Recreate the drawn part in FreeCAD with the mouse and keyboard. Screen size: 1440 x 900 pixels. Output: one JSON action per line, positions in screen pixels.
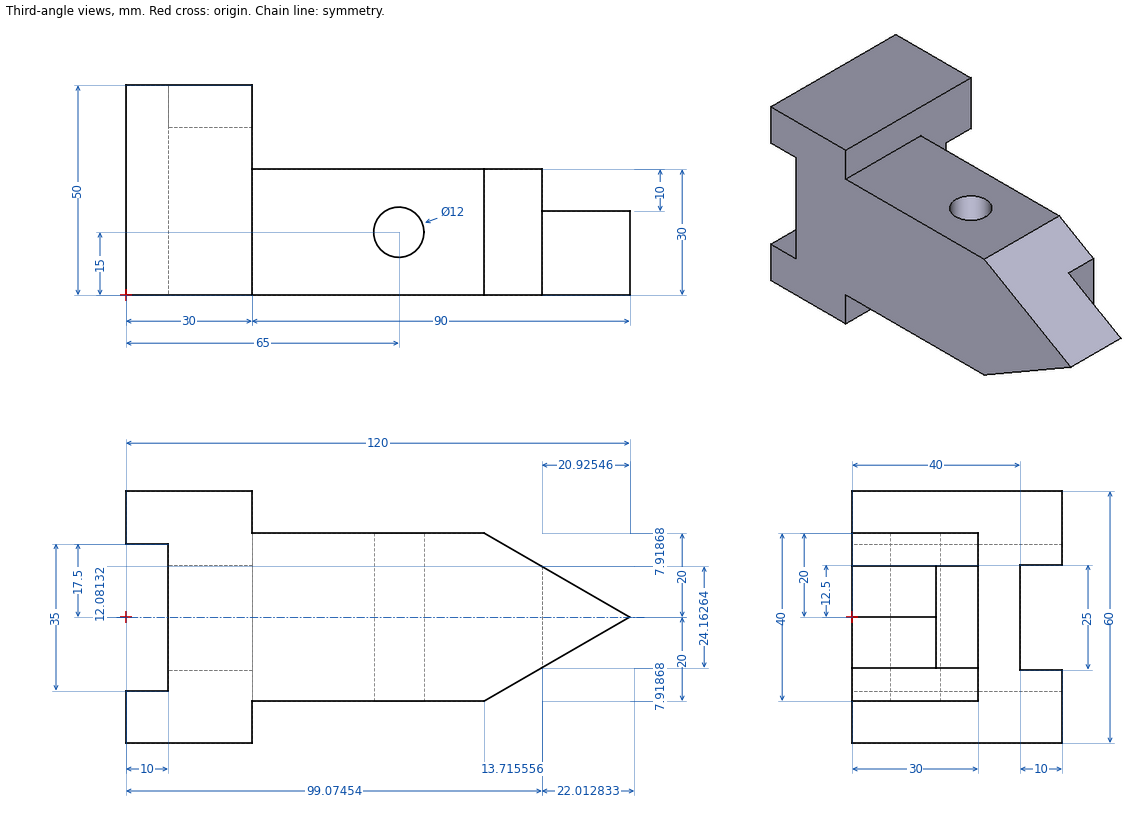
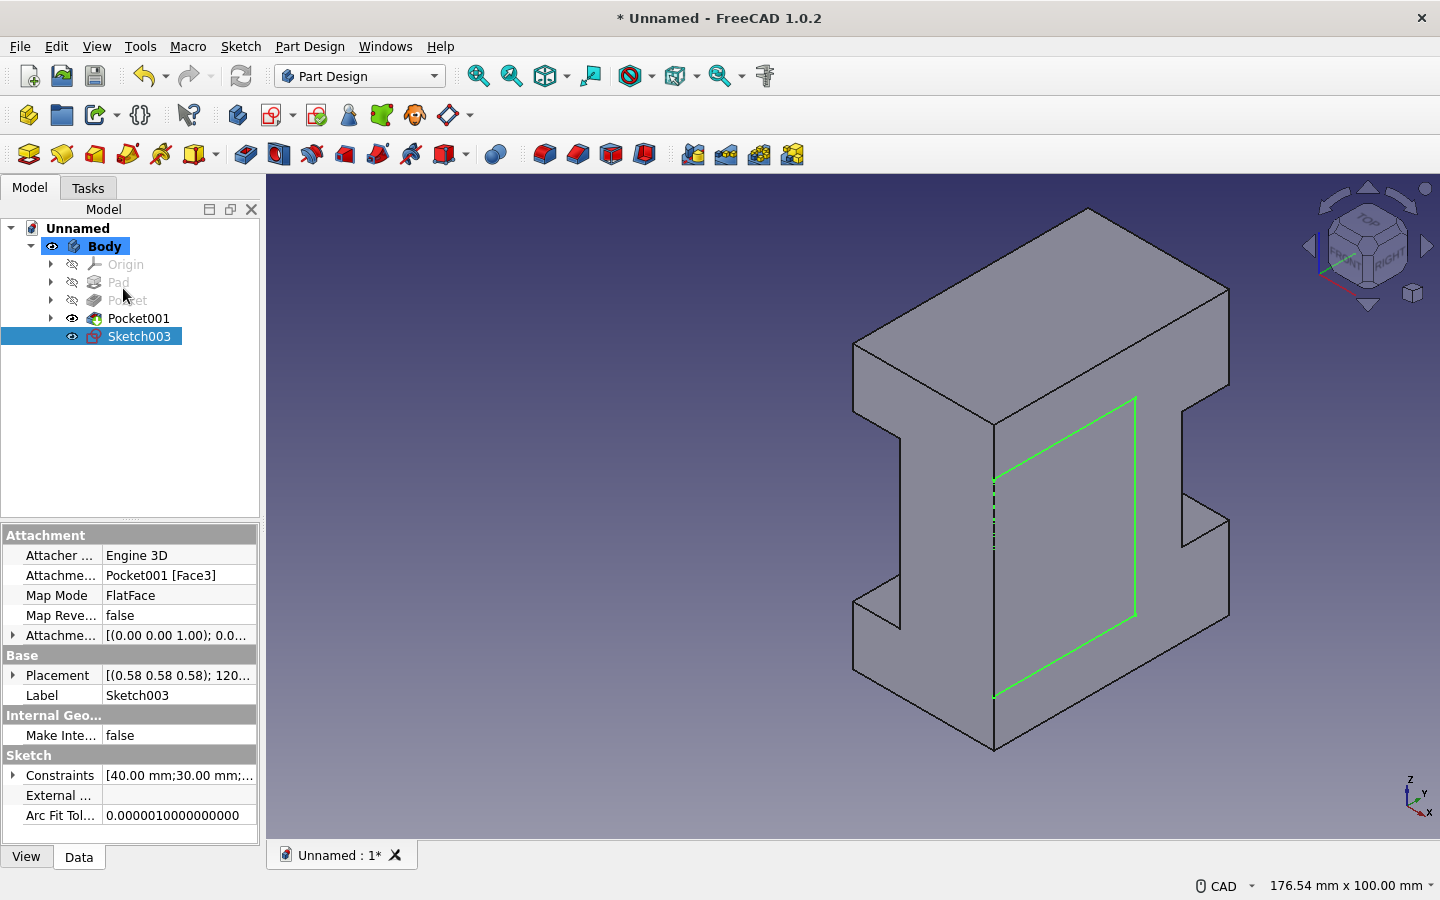
{"action": "left_click", "coordinate": [29, 154]}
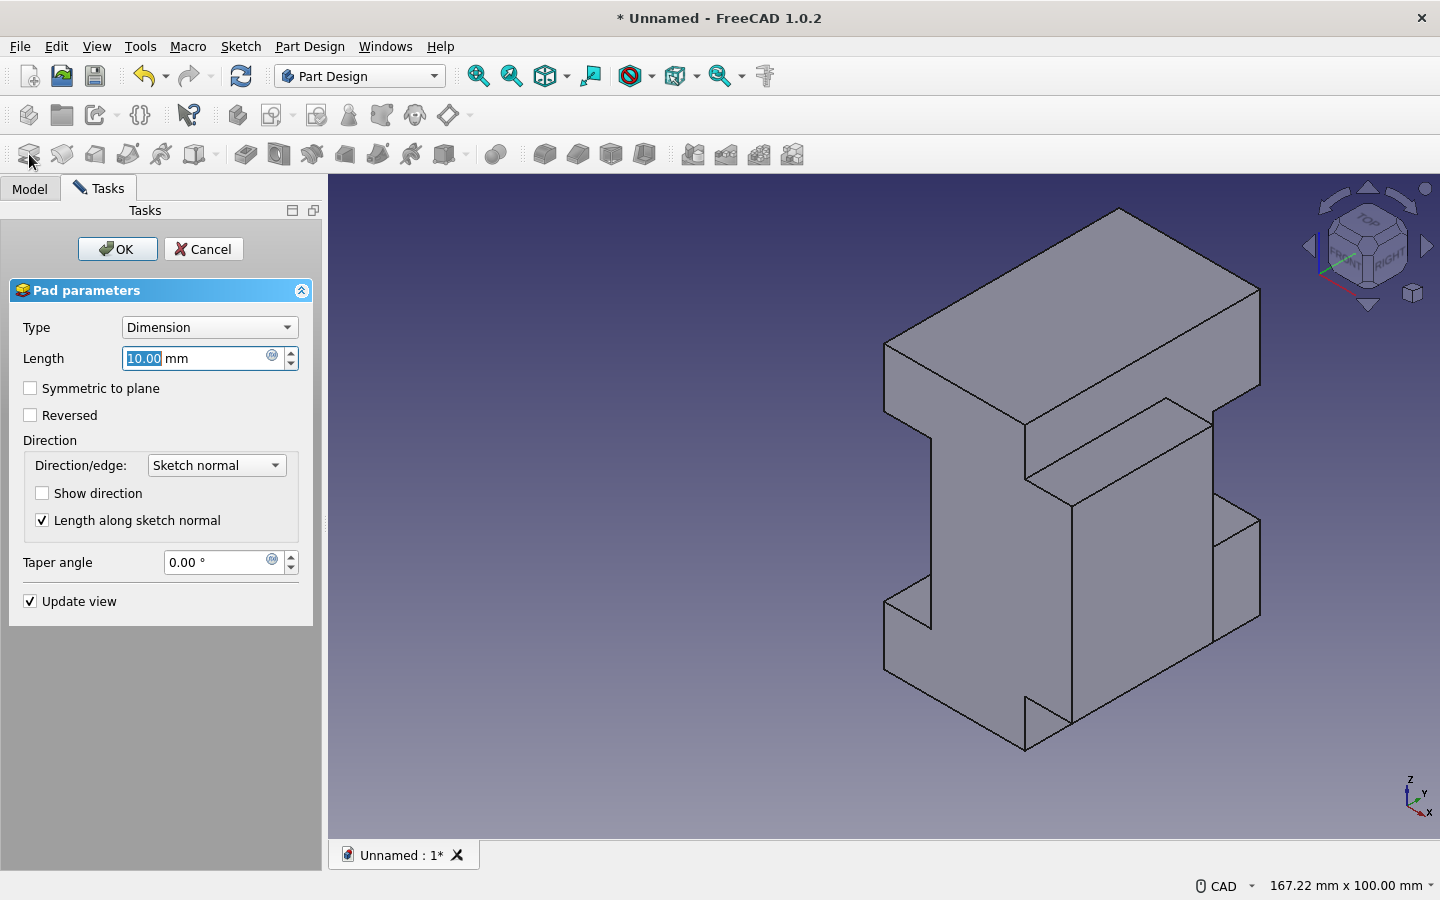
{"action": "type", "text": "90"}
{"action": "key", "text": "Tab"}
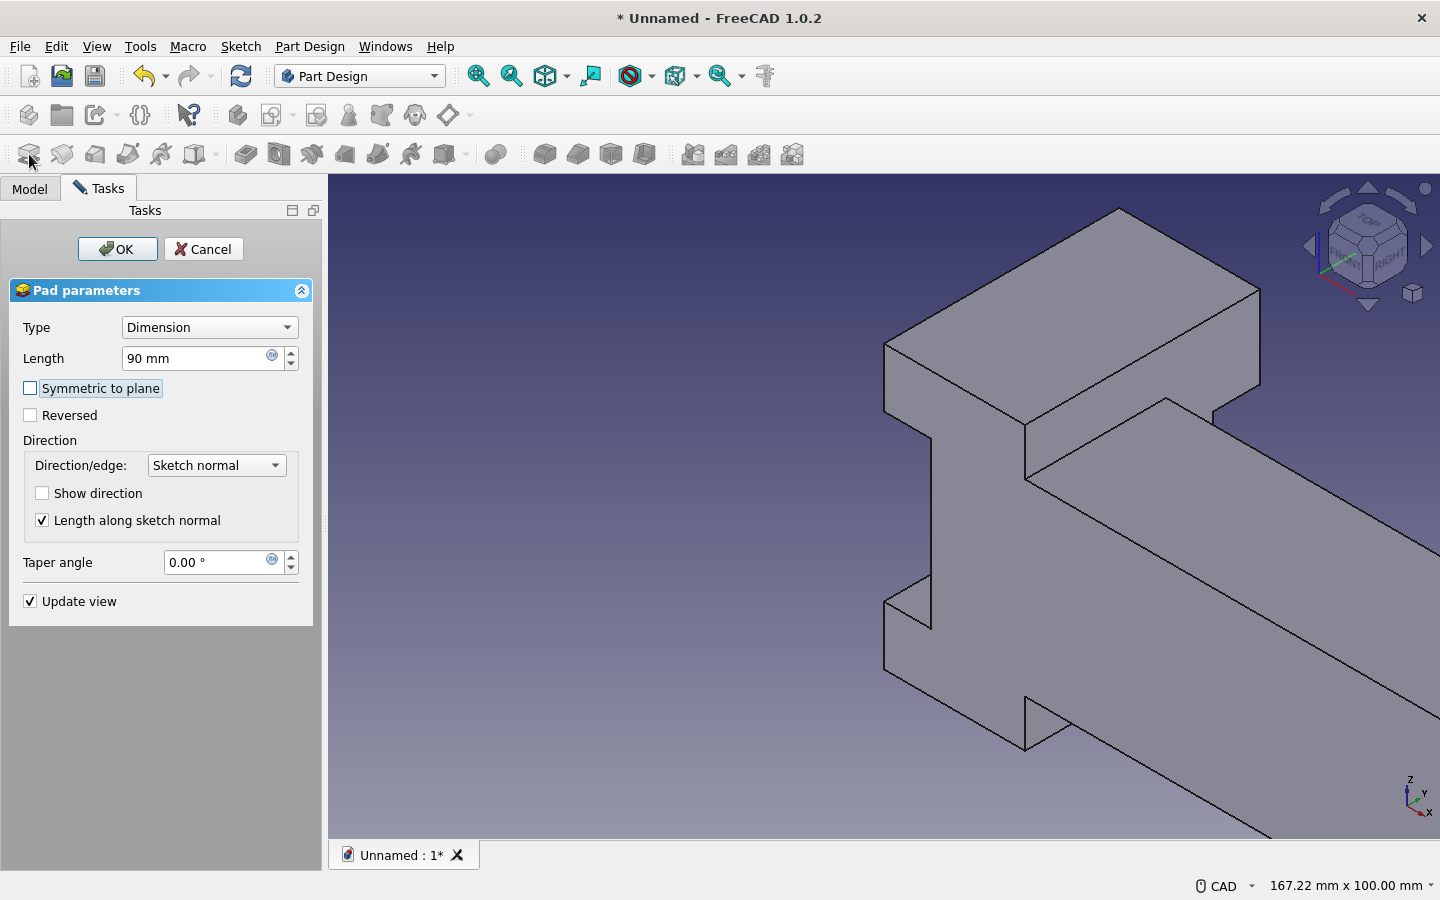
{"action": "left_click", "coordinate": [118, 249]}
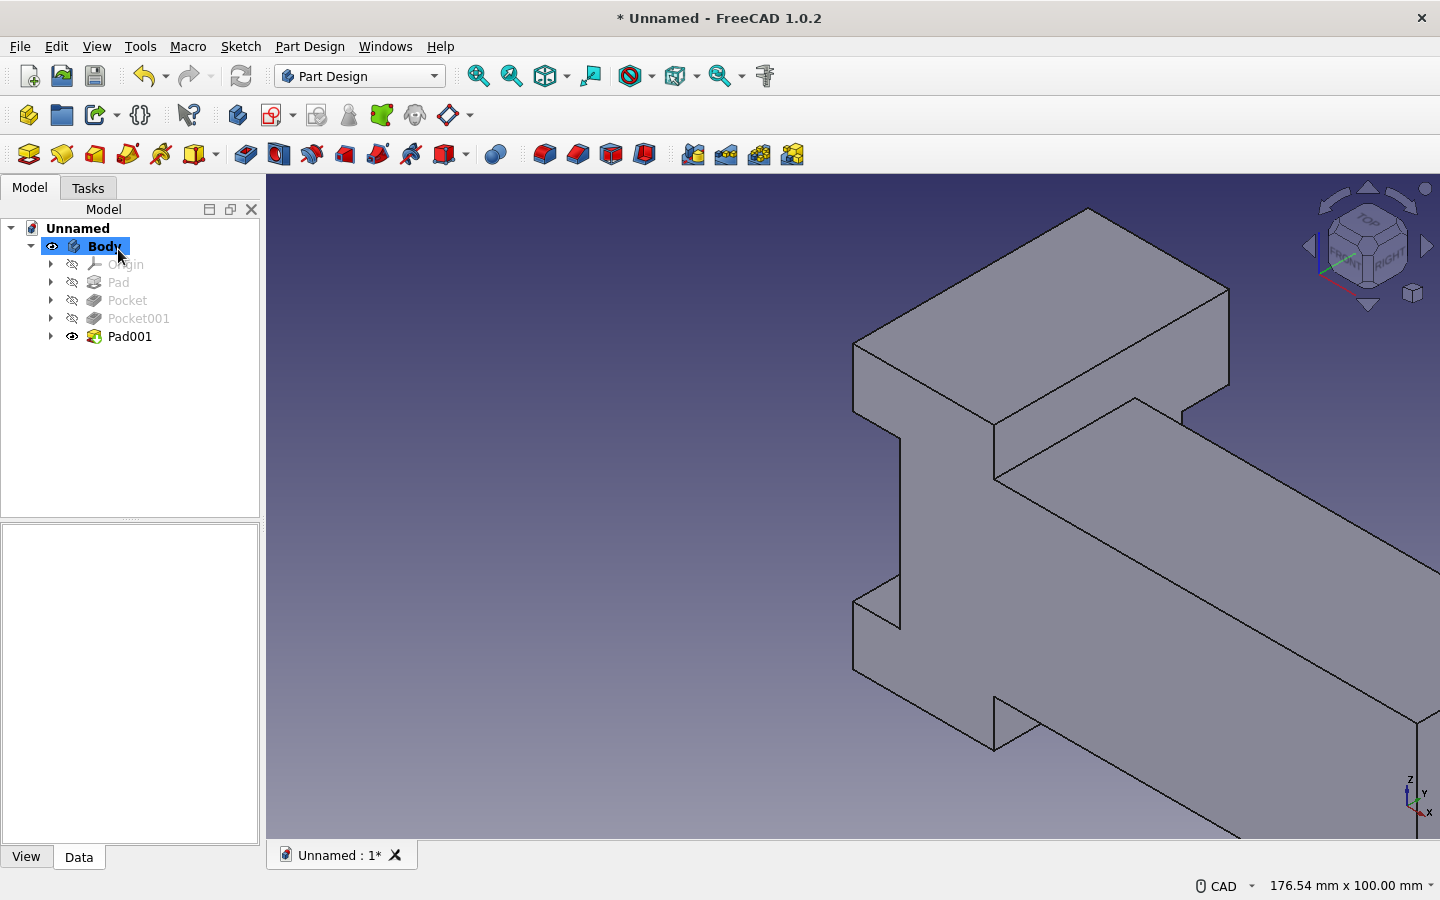
{"action": "left_click", "coordinate": [479, 76]}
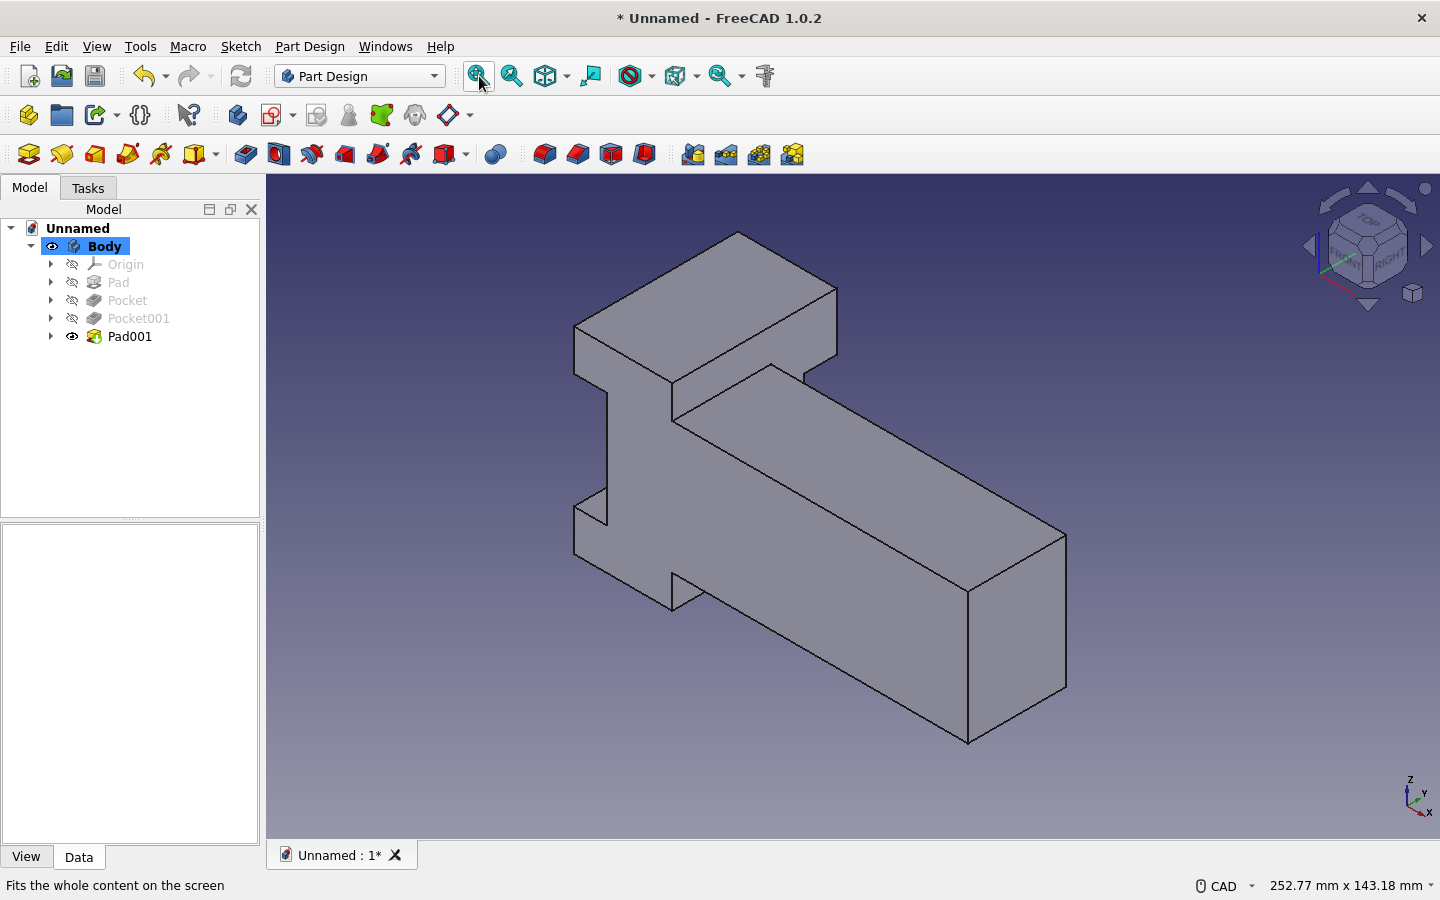
{"action": "left_click", "coordinate": [954, 526]}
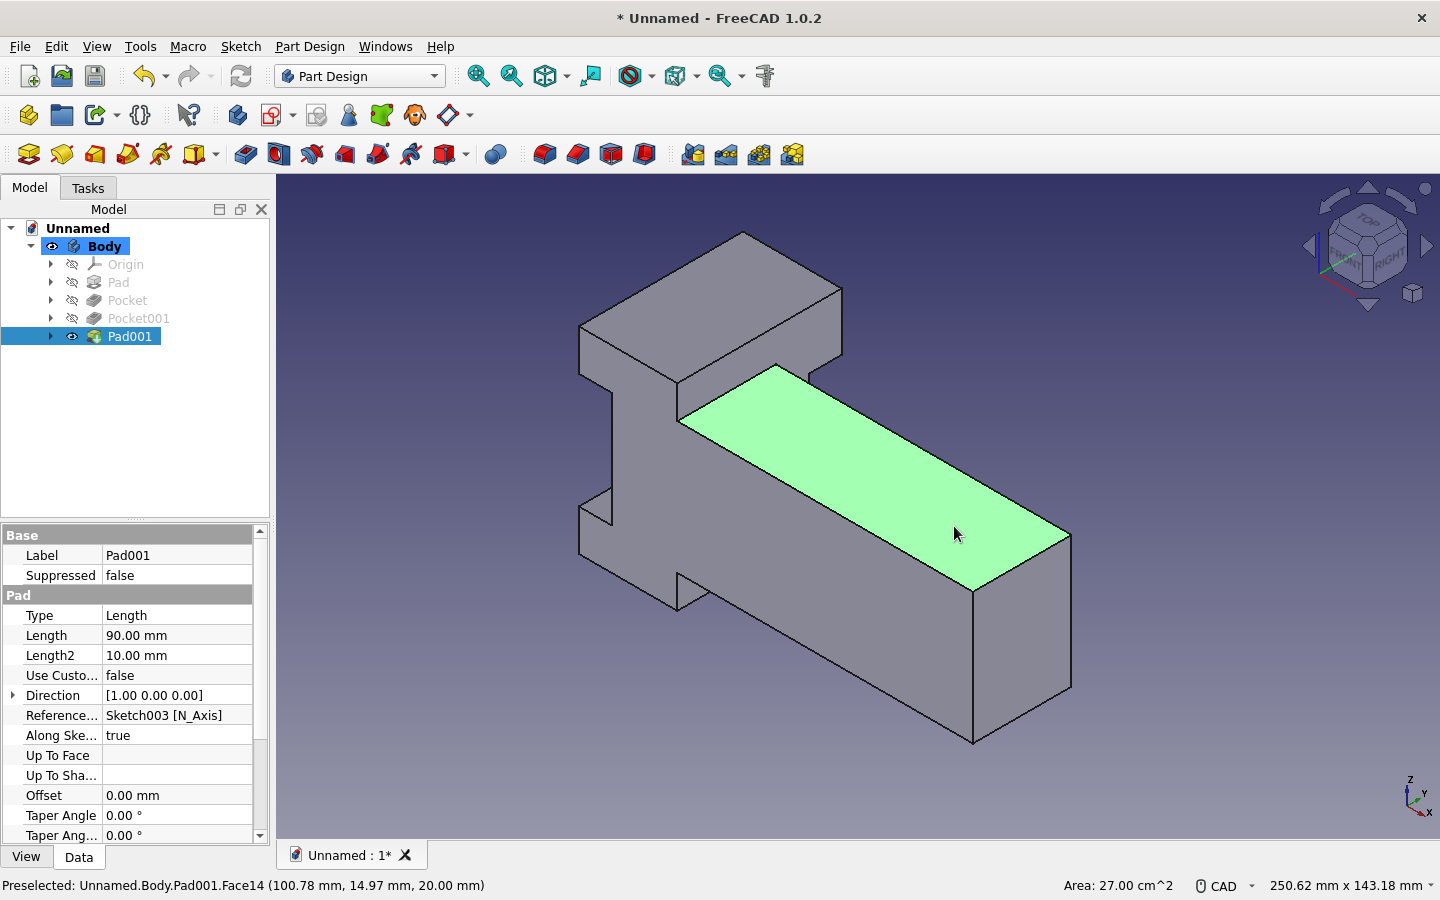
{"action": "left_click", "coordinate": [270, 116]}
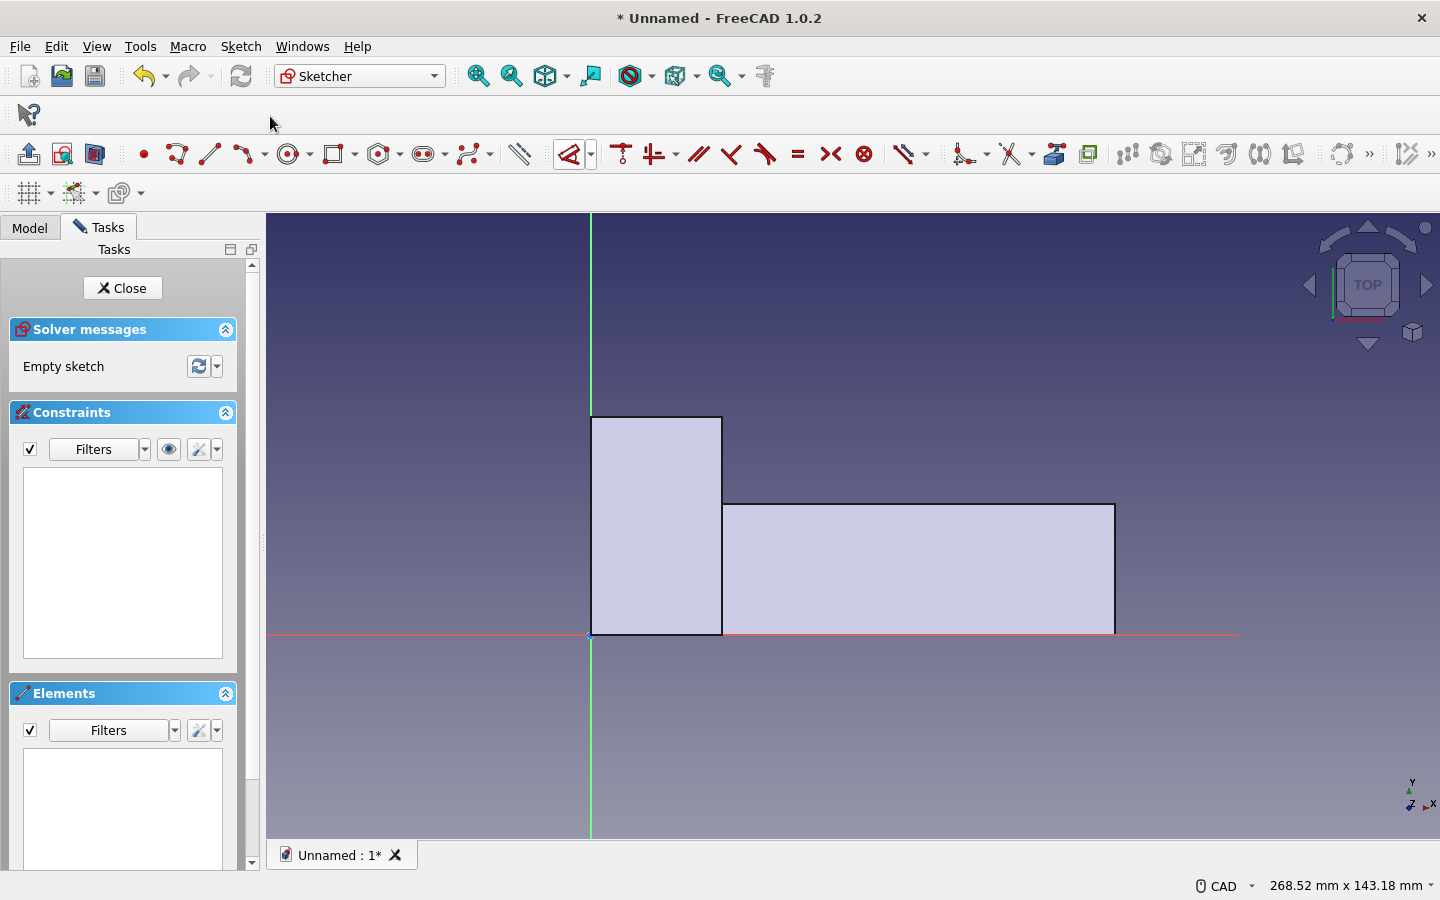
{"action": "scroll", "coordinate": [889, 577], "scroll_direction": "up", "scroll_amount": 10}